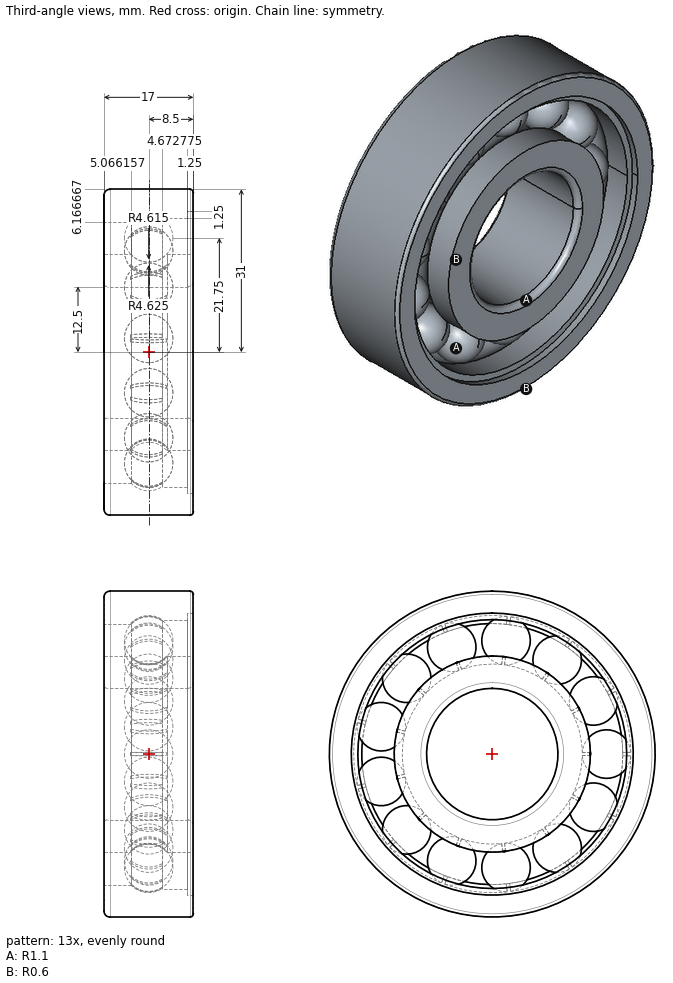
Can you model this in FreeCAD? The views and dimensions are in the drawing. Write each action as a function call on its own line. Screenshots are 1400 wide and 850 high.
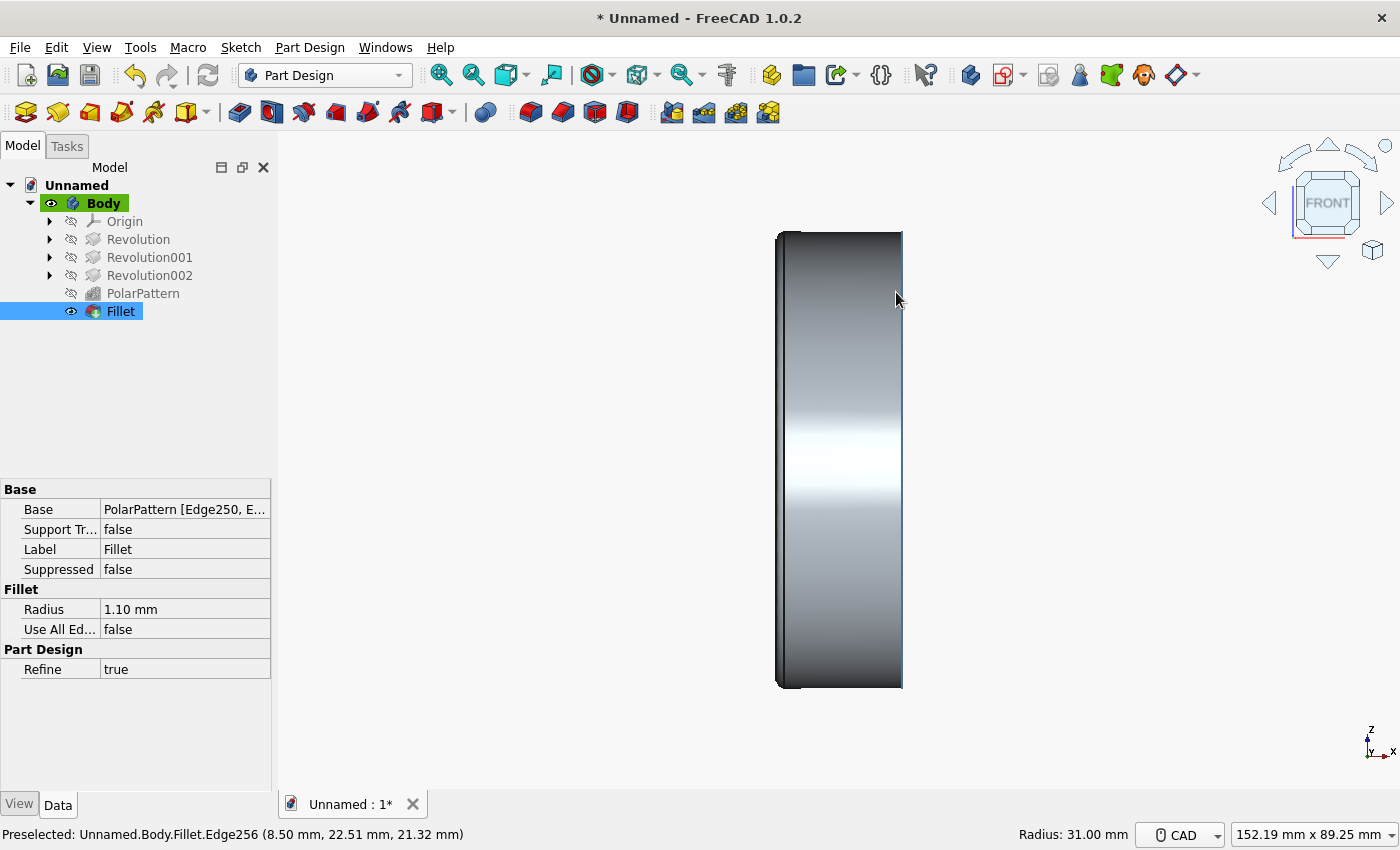
key(3)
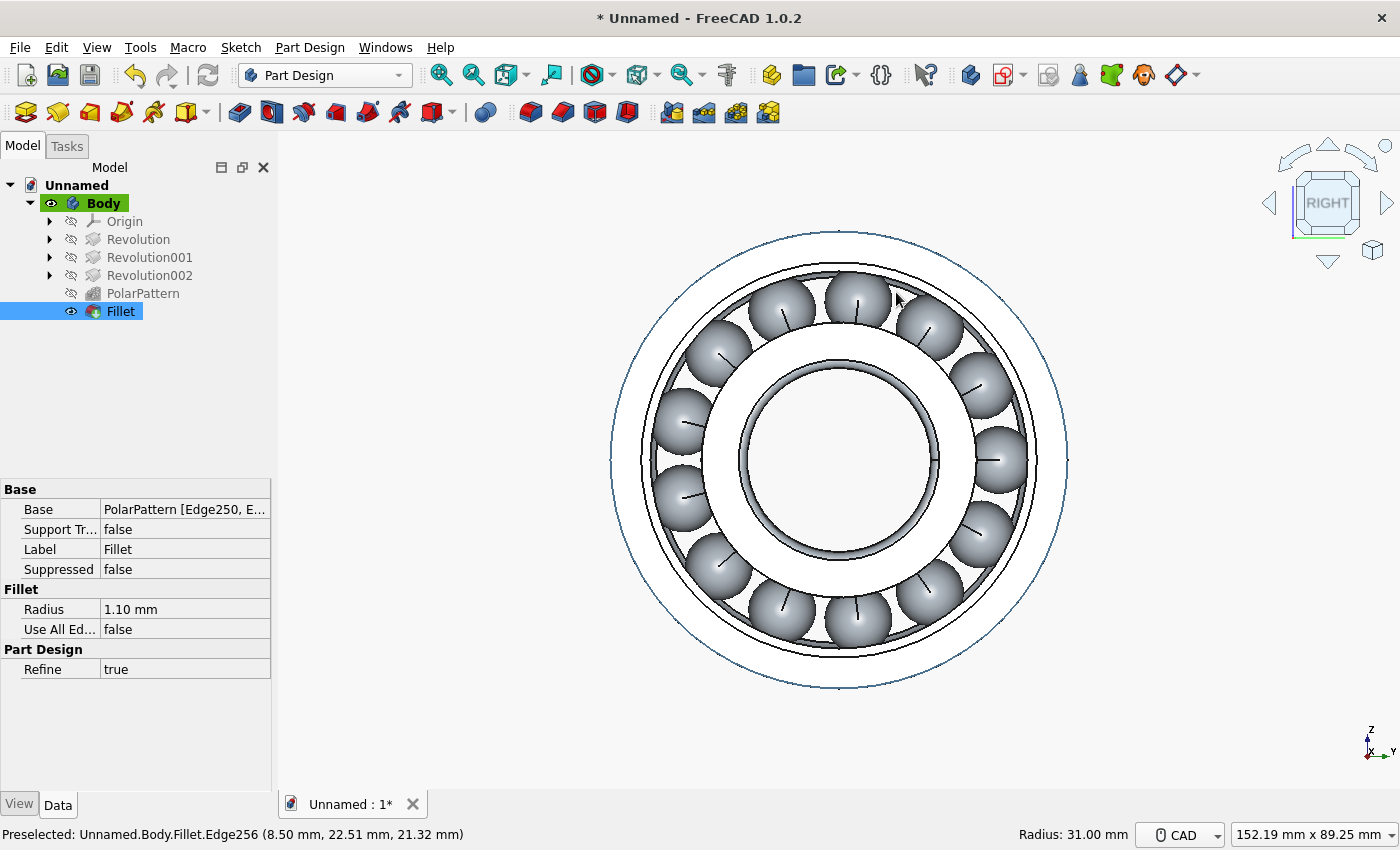
key(5)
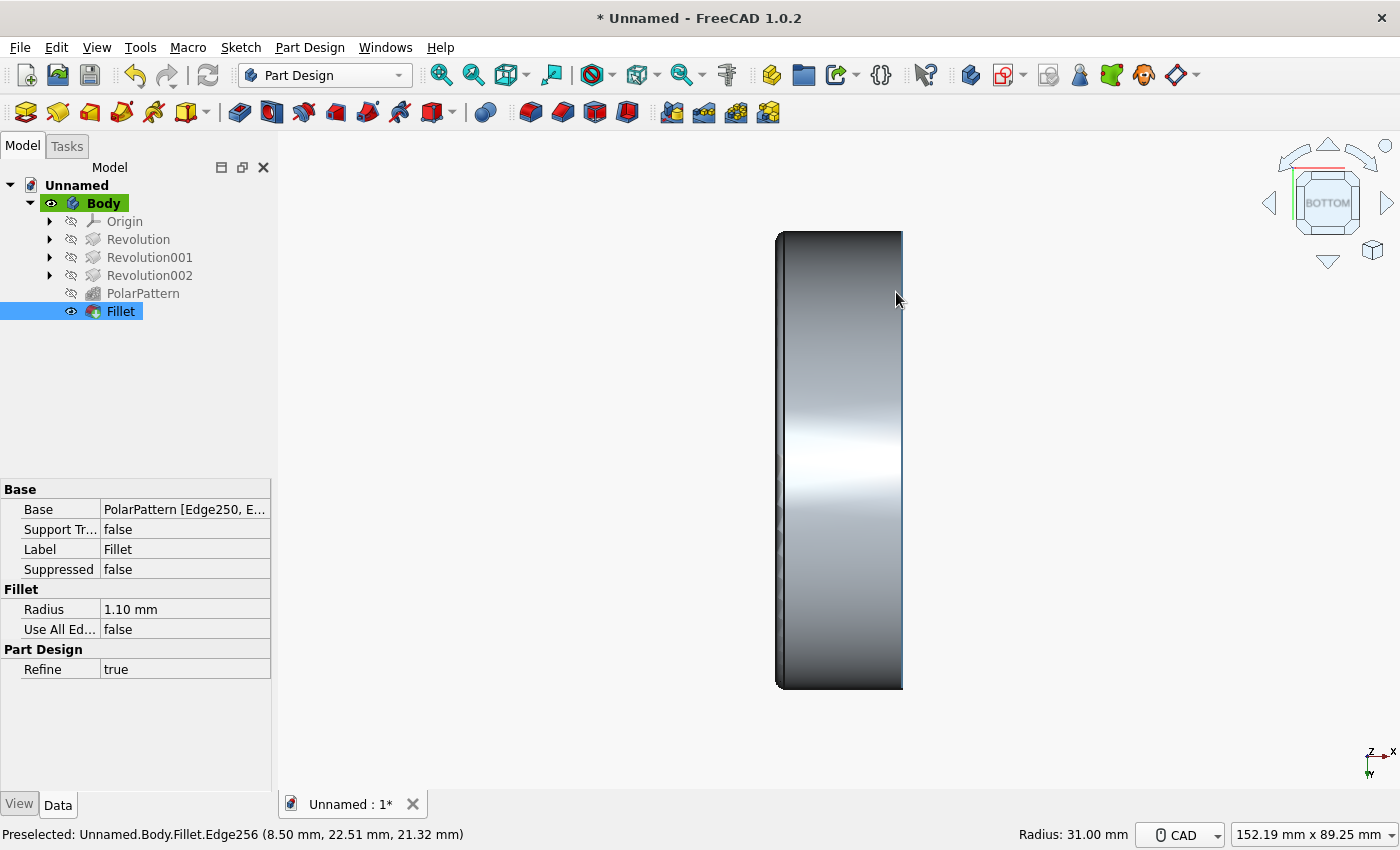
key(4)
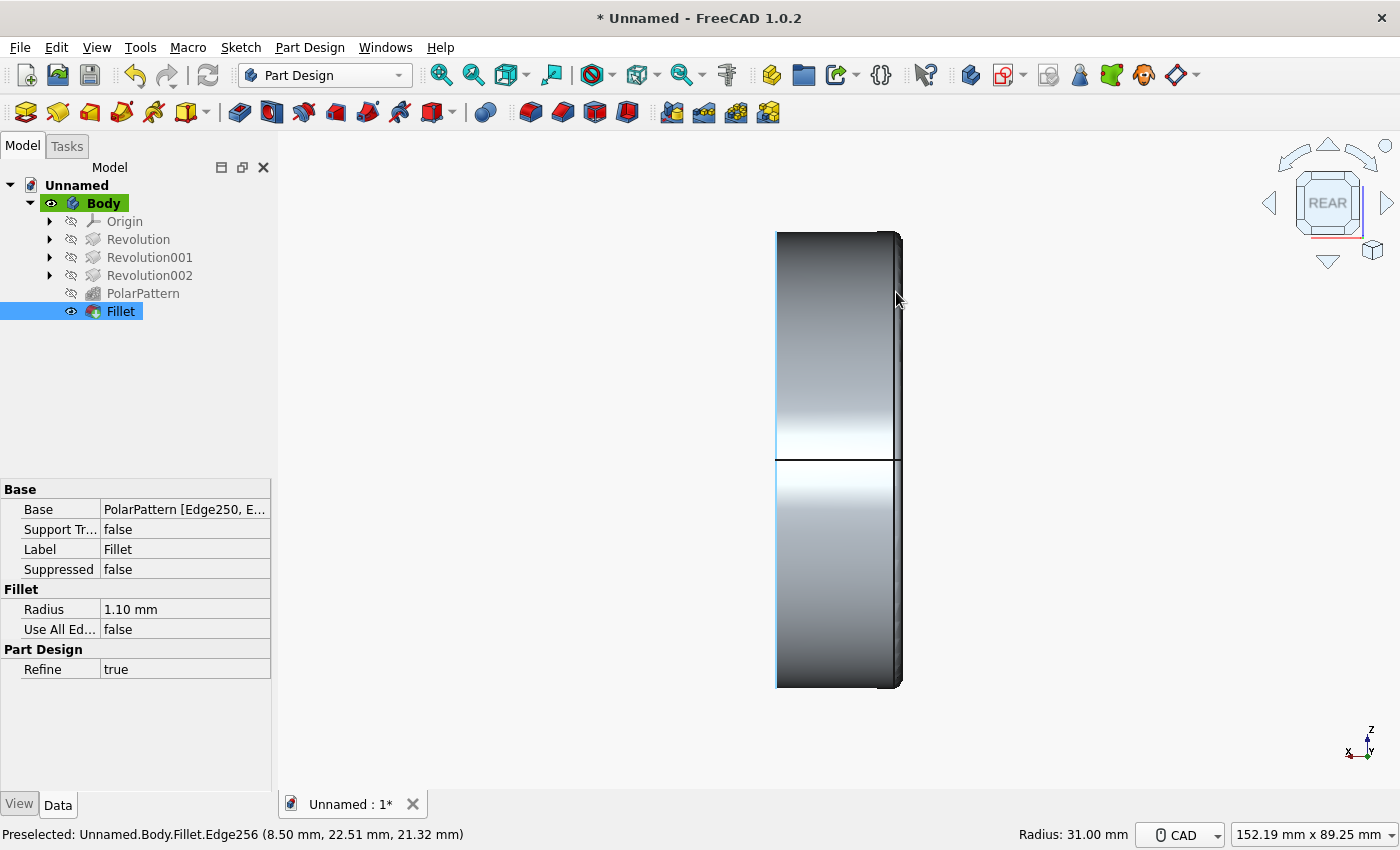
key(6)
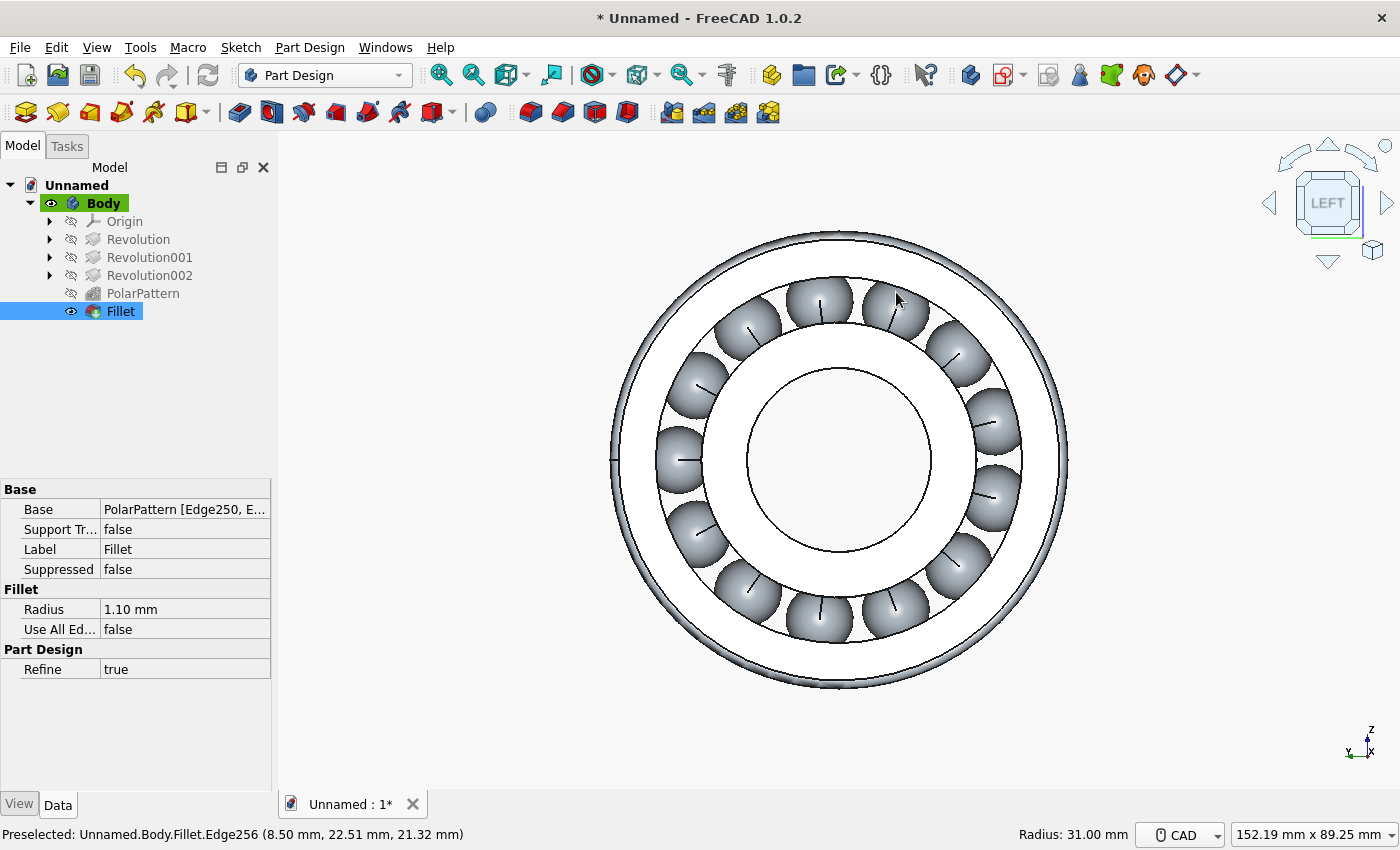
click(931, 459, ctrl)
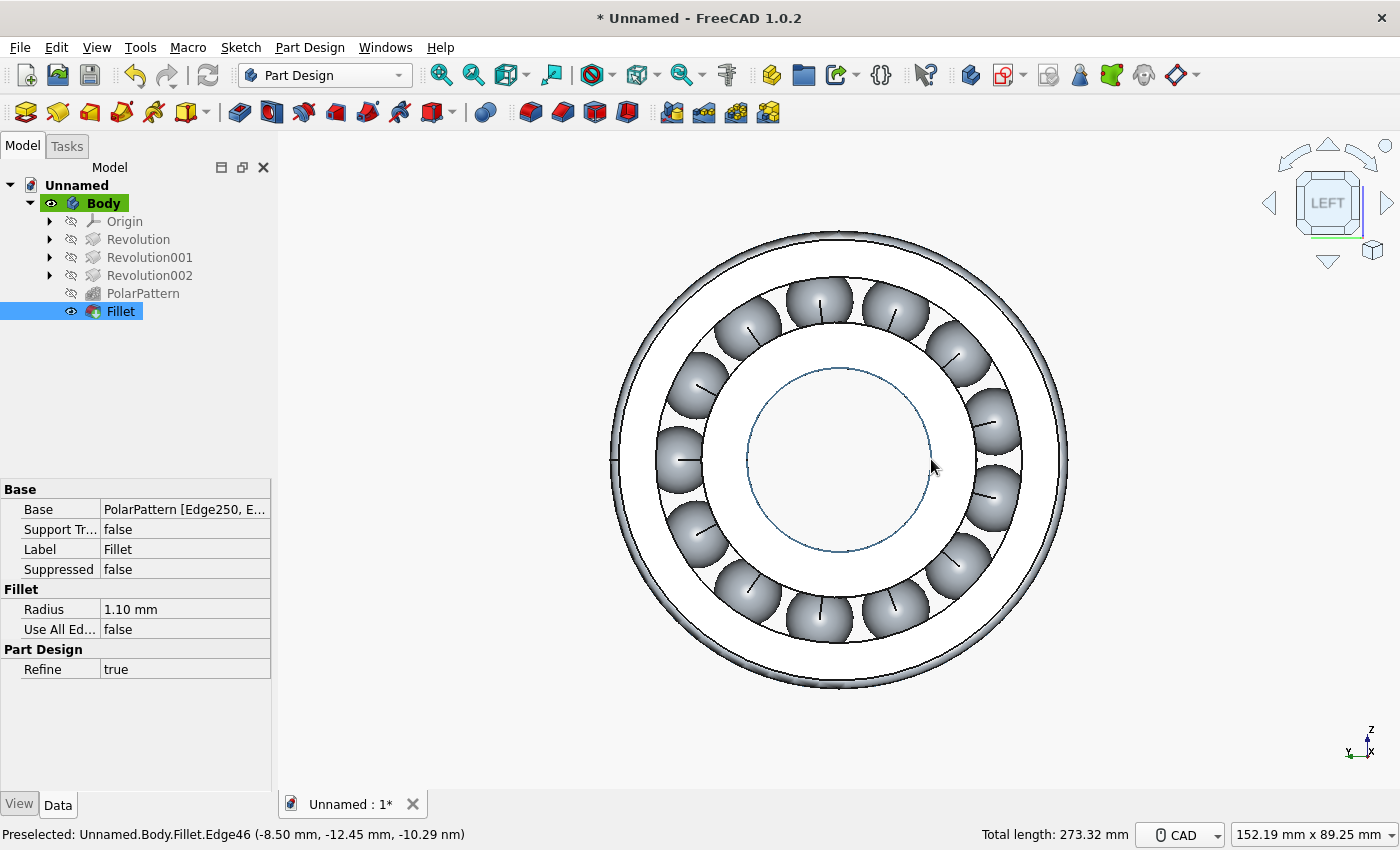
click(532, 112)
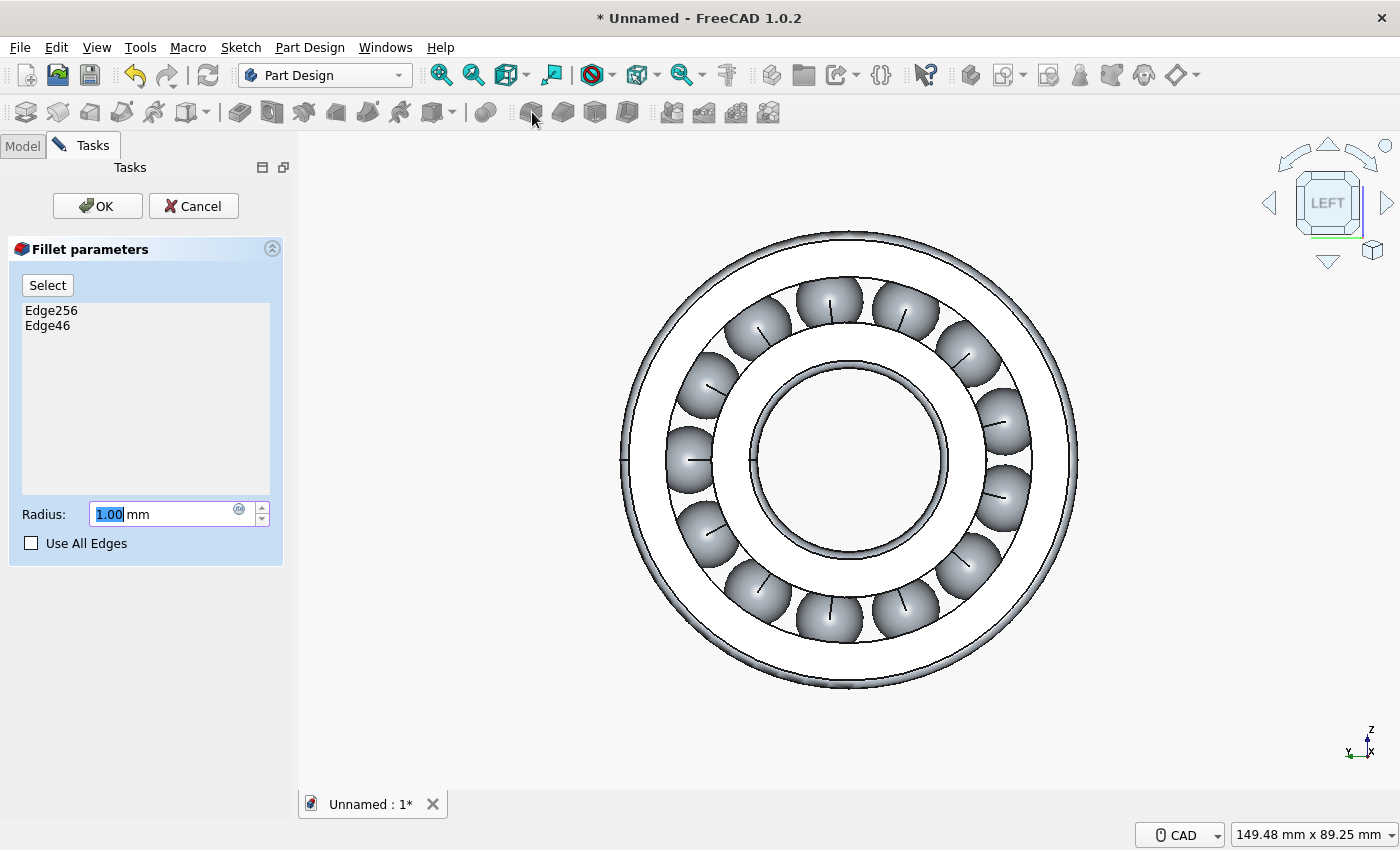
text(0.6)
key(Tab)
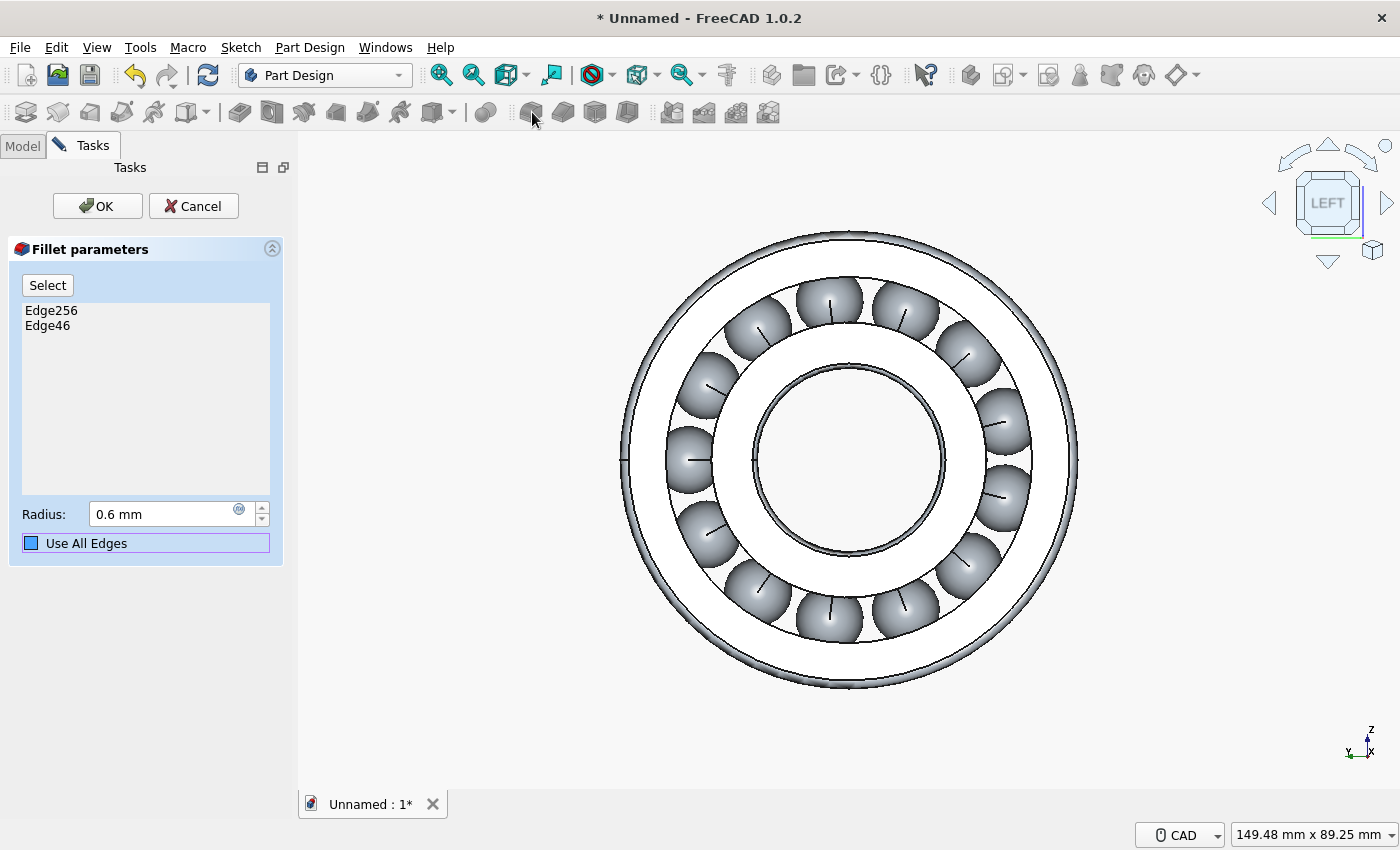
click(98, 206)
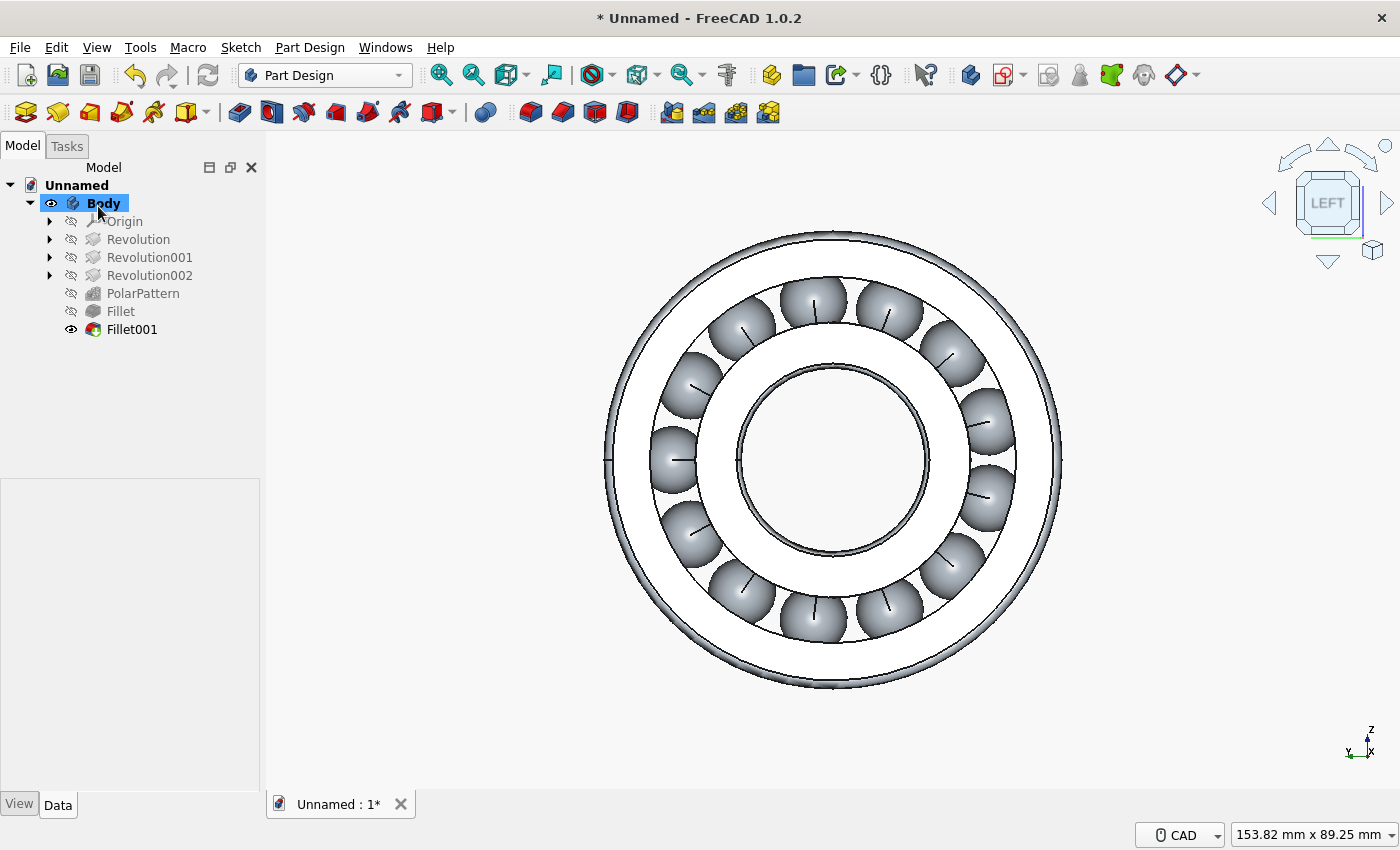
key(0)